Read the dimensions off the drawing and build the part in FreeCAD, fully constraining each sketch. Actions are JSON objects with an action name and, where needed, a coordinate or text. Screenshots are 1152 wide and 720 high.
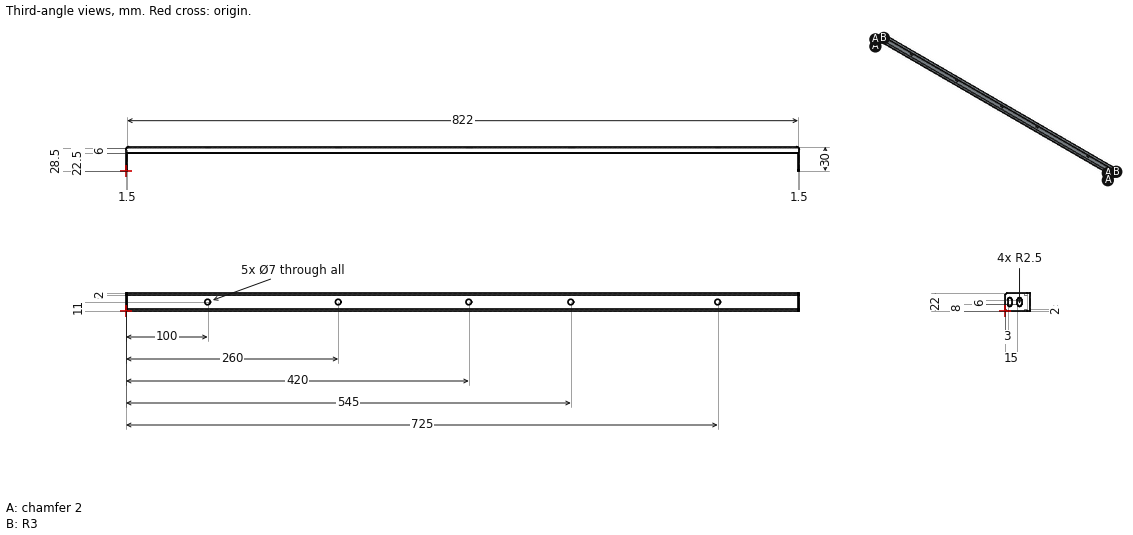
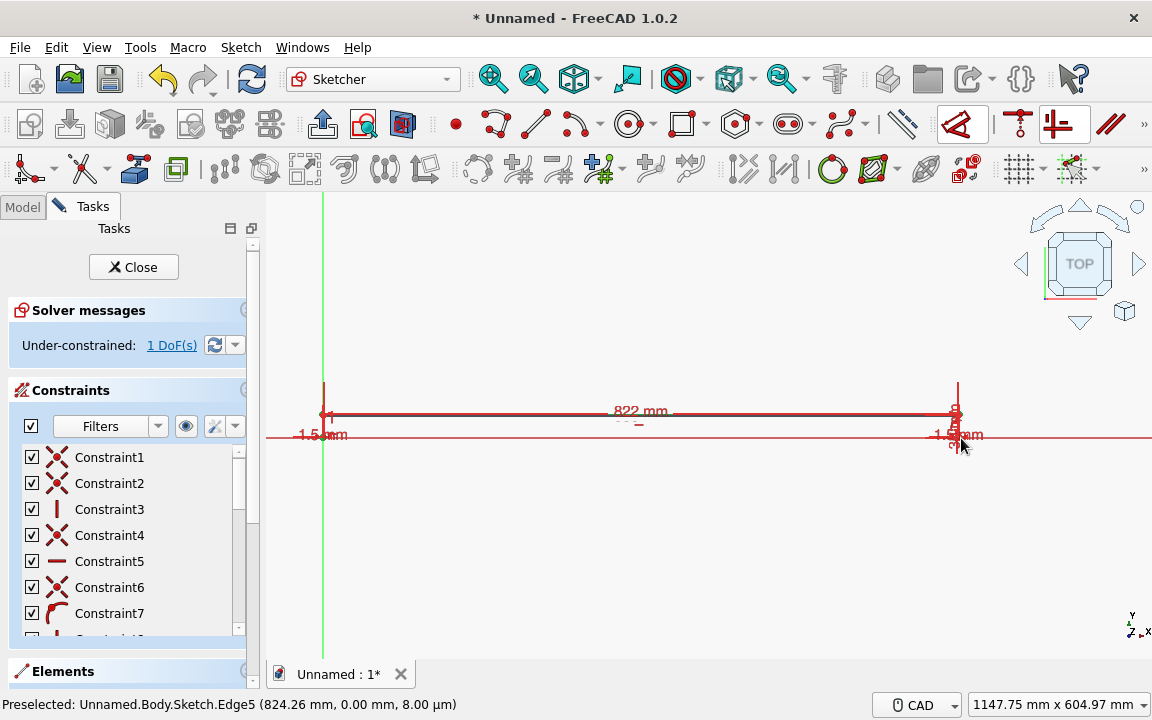
{"action": "scroll", "coordinate": [324, 431], "scroll_direction": "up", "scroll_amount": 13}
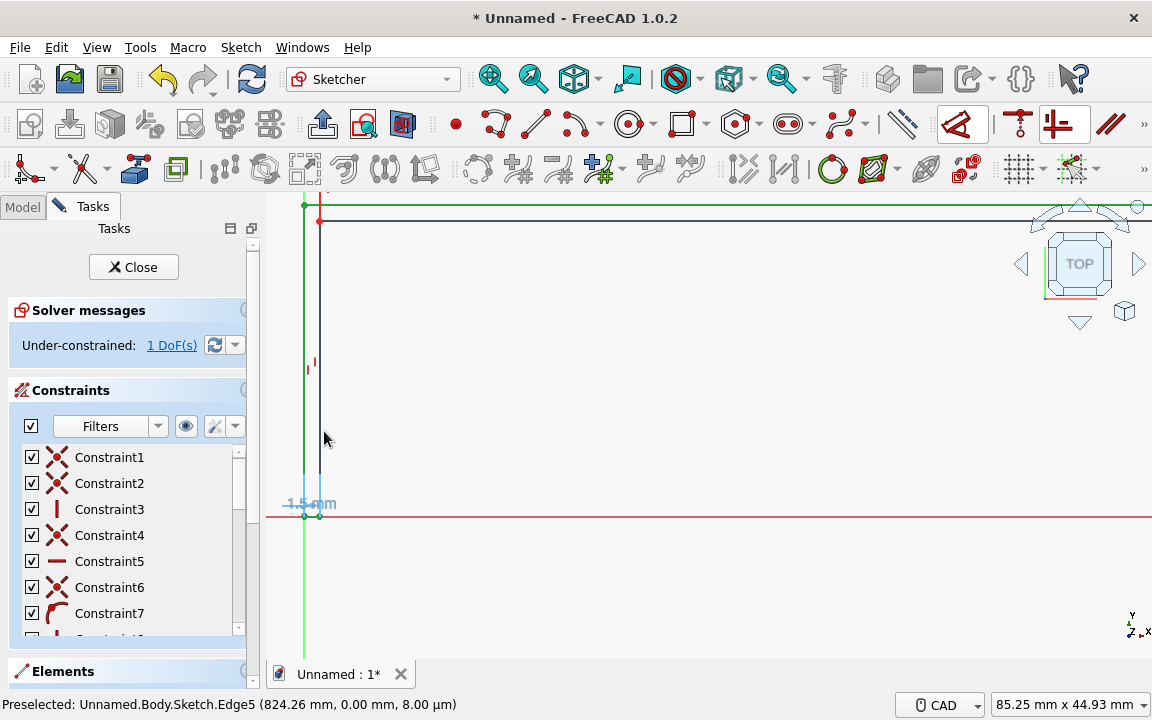
{"action": "left_click", "coordinate": [320, 428]}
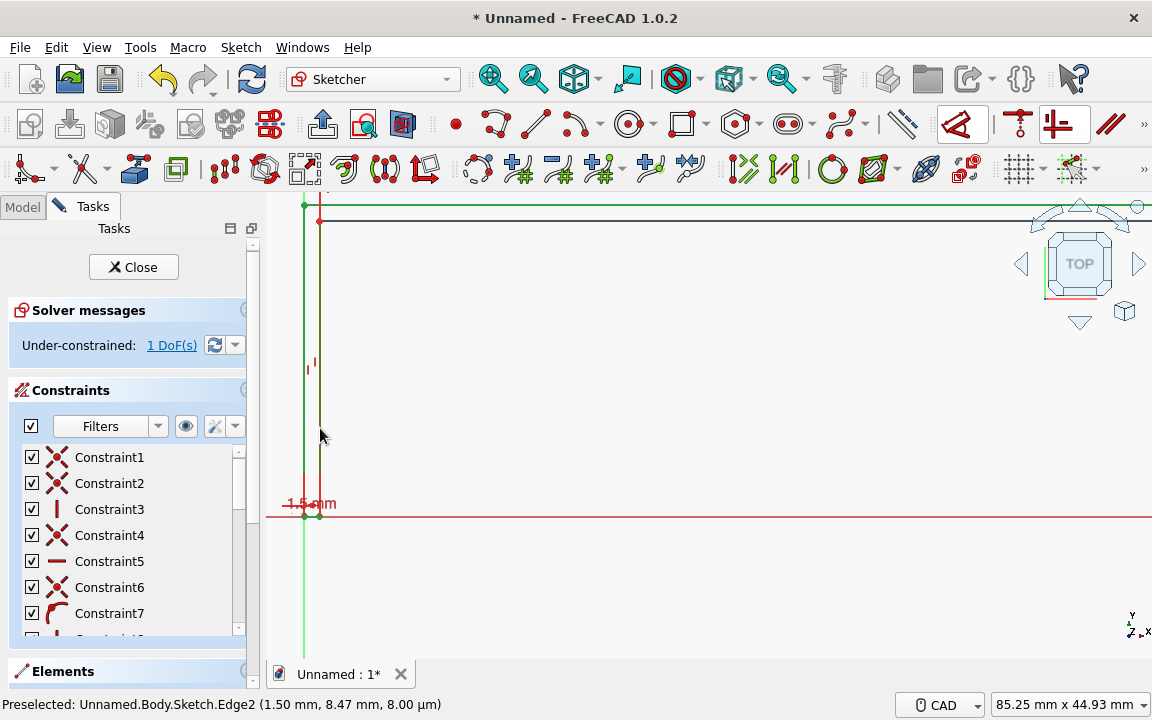
{"action": "left_click", "coordinate": [982, 124]}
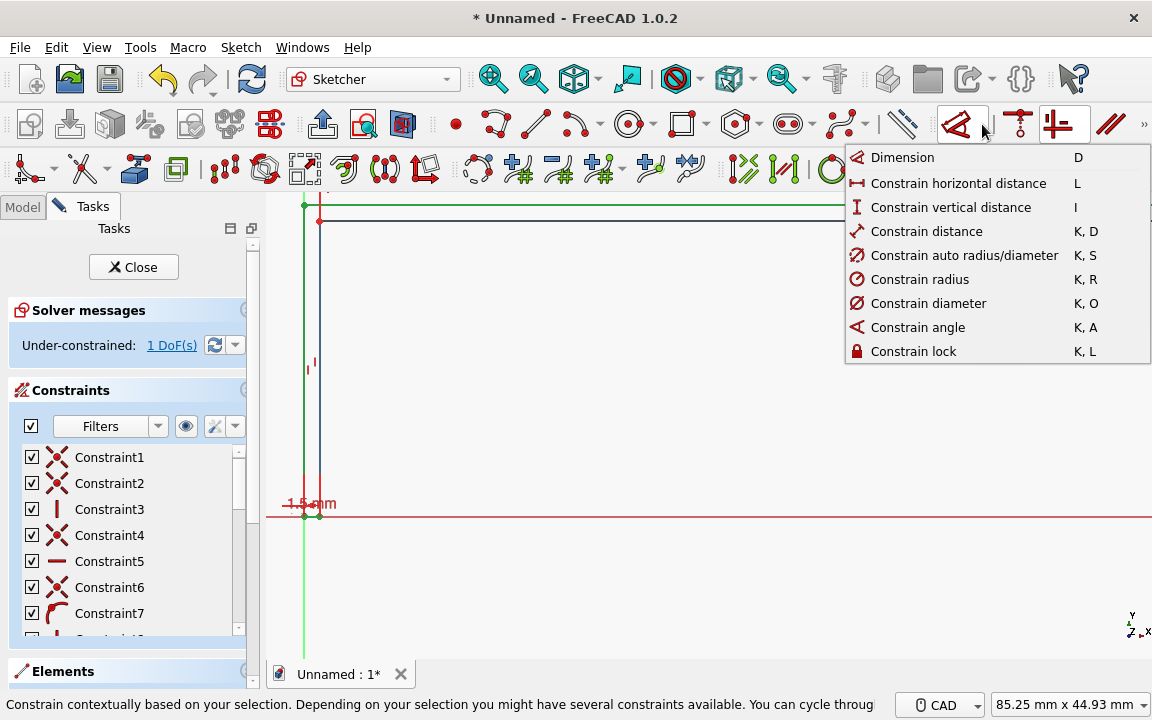
{"action": "left_click", "coordinate": [998, 207]}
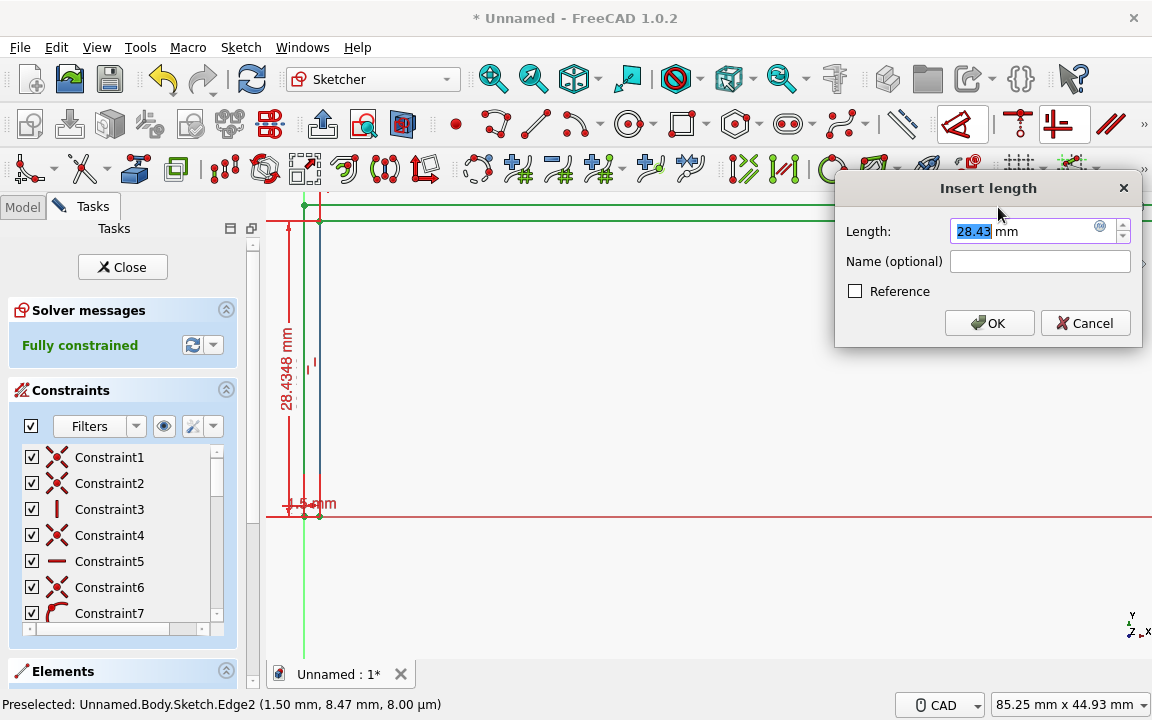
{"action": "type", "text": "28.5"}
{"action": "key", "text": "Return"}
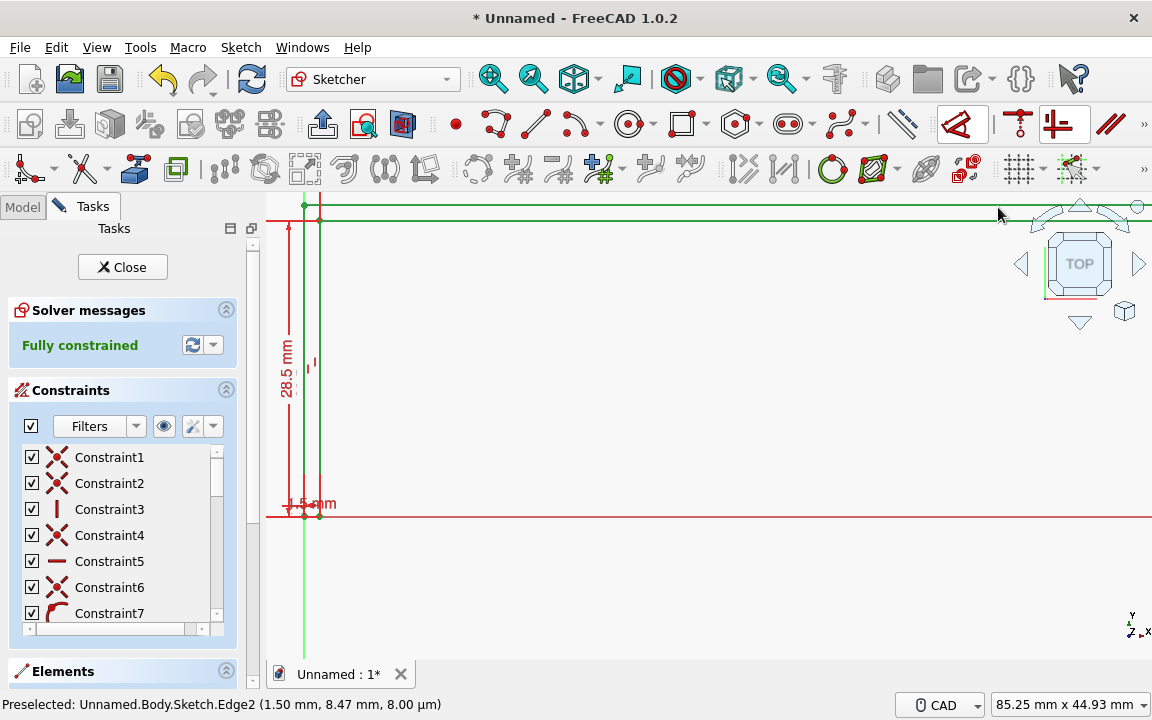
{"action": "left_click", "coordinate": [123, 267]}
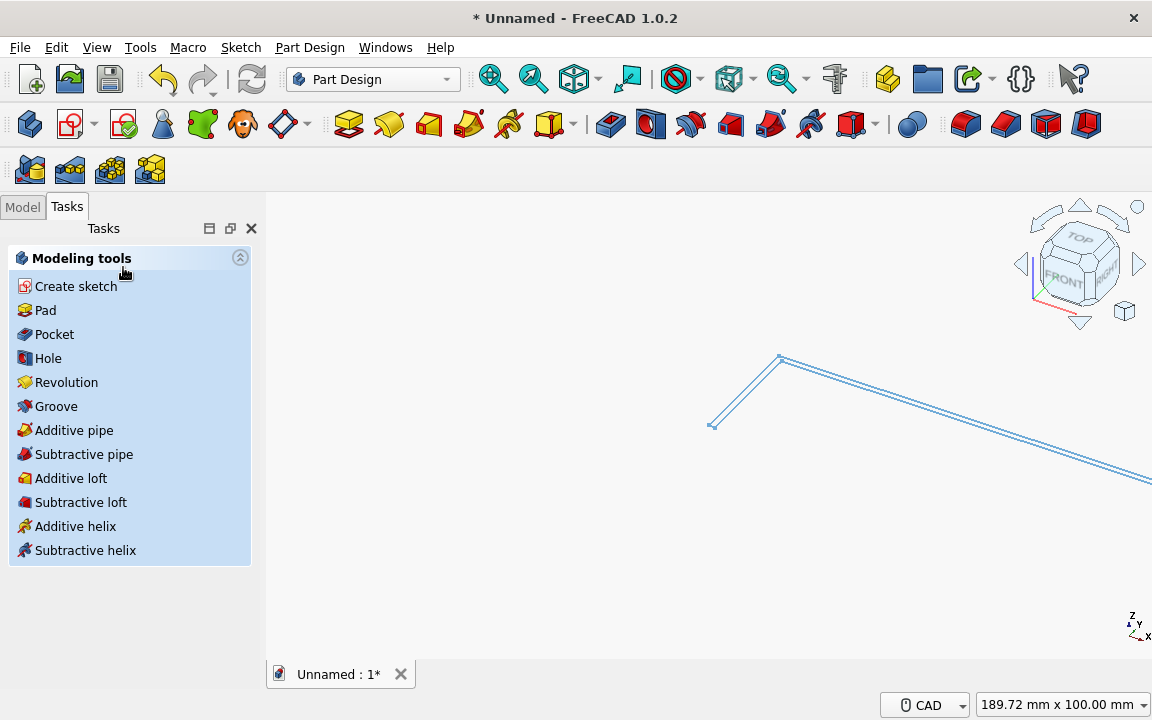
{"action": "left_click", "coordinate": [350, 124]}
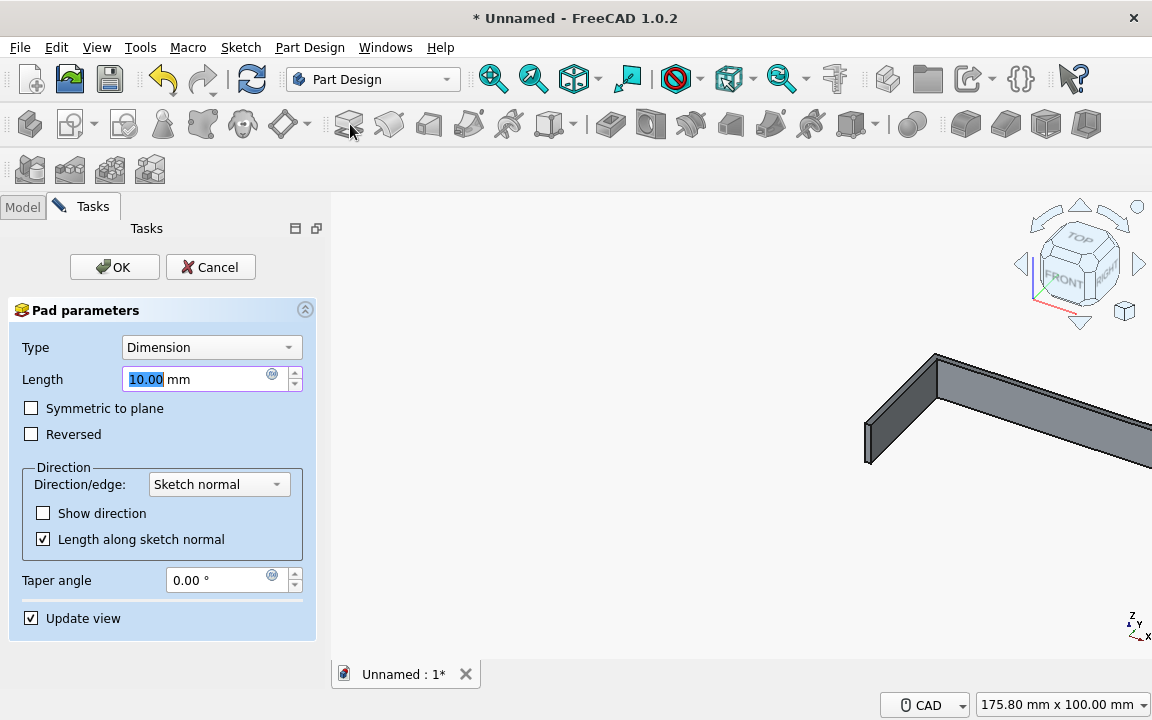
{"action": "type", "text": "22"}
{"action": "key", "text": "Tab"}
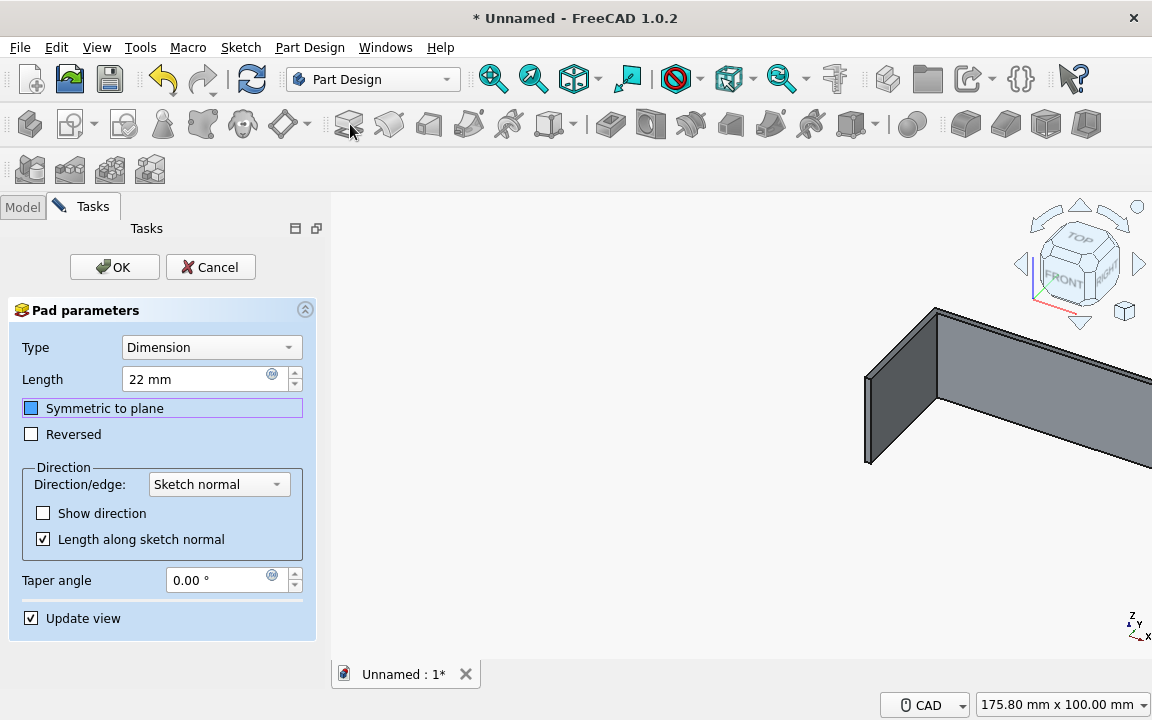
{"action": "left_click", "coordinate": [115, 267]}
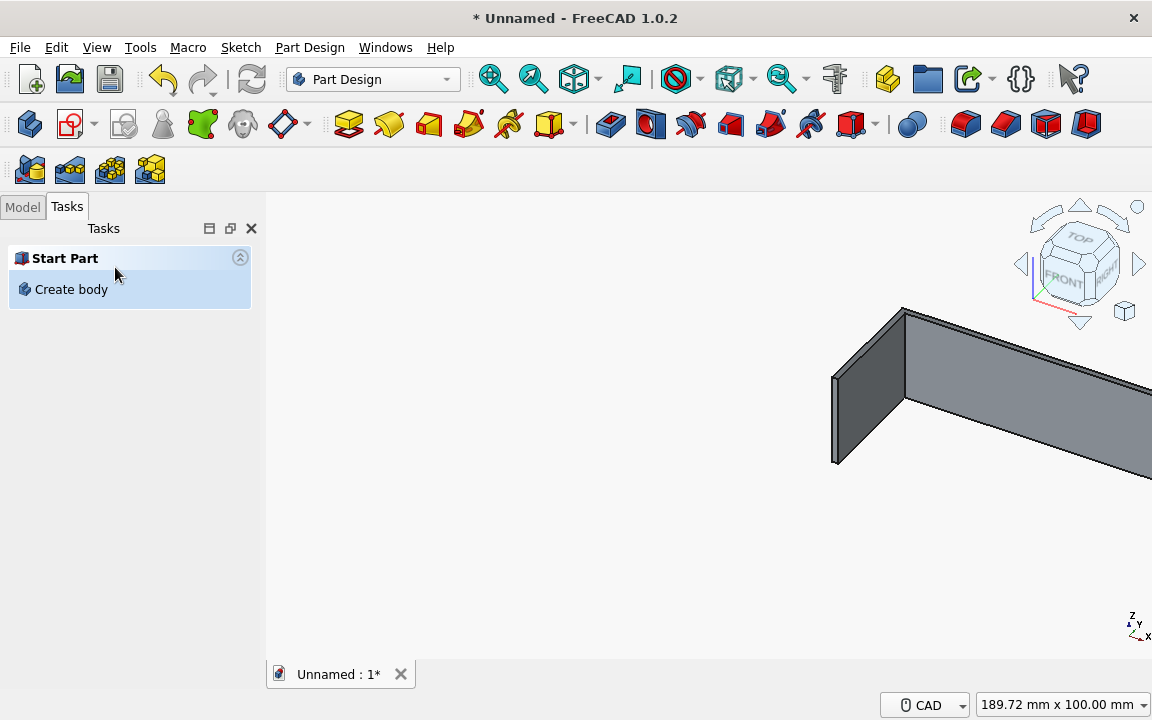
{"action": "left_click", "coordinate": [494, 80]}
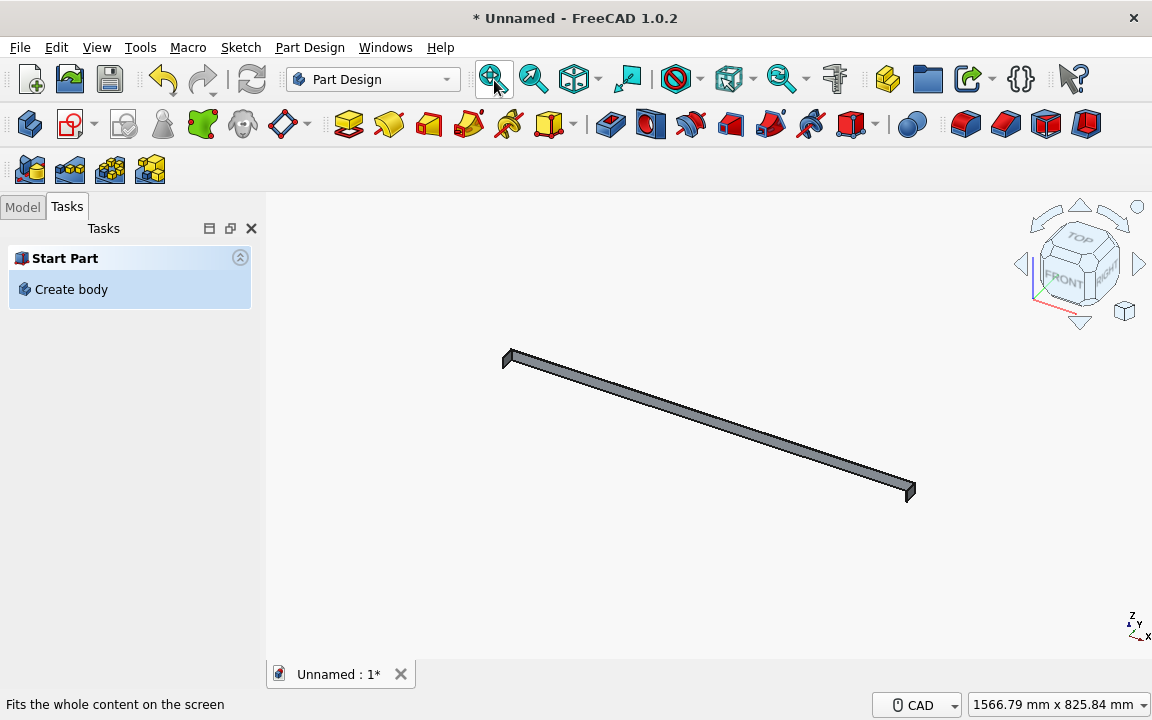
{"action": "scroll", "coordinate": [912, 485], "scroll_direction": "up", "scroll_amount": 15}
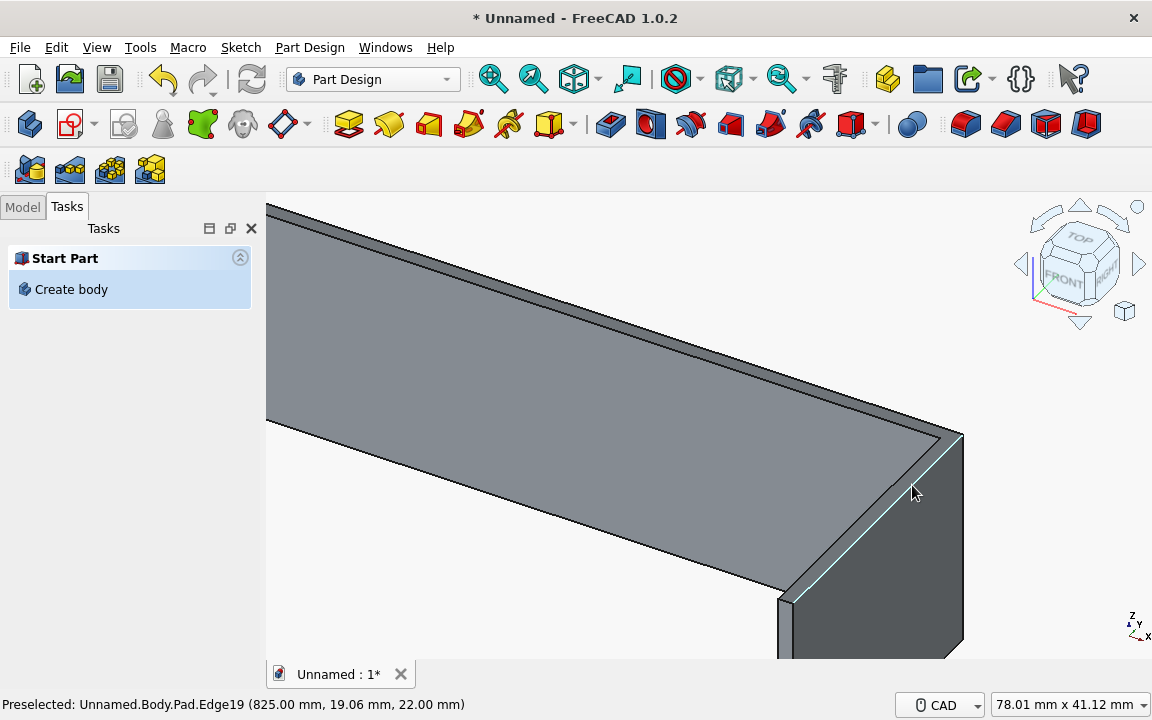
{"action": "left_click", "coordinate": [837, 546]}